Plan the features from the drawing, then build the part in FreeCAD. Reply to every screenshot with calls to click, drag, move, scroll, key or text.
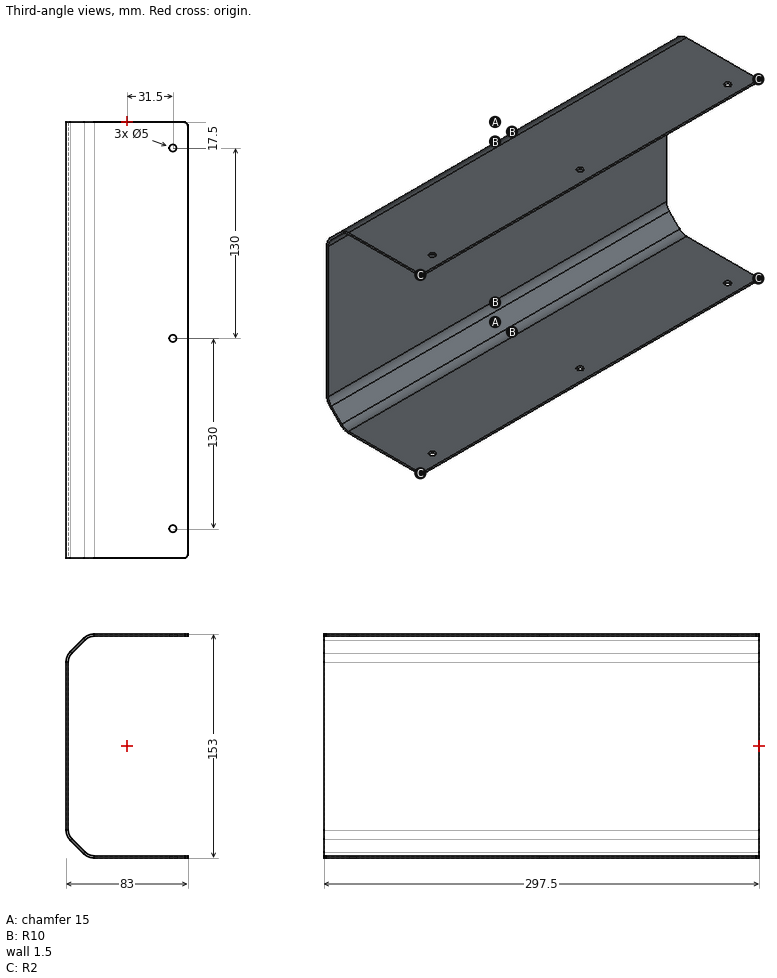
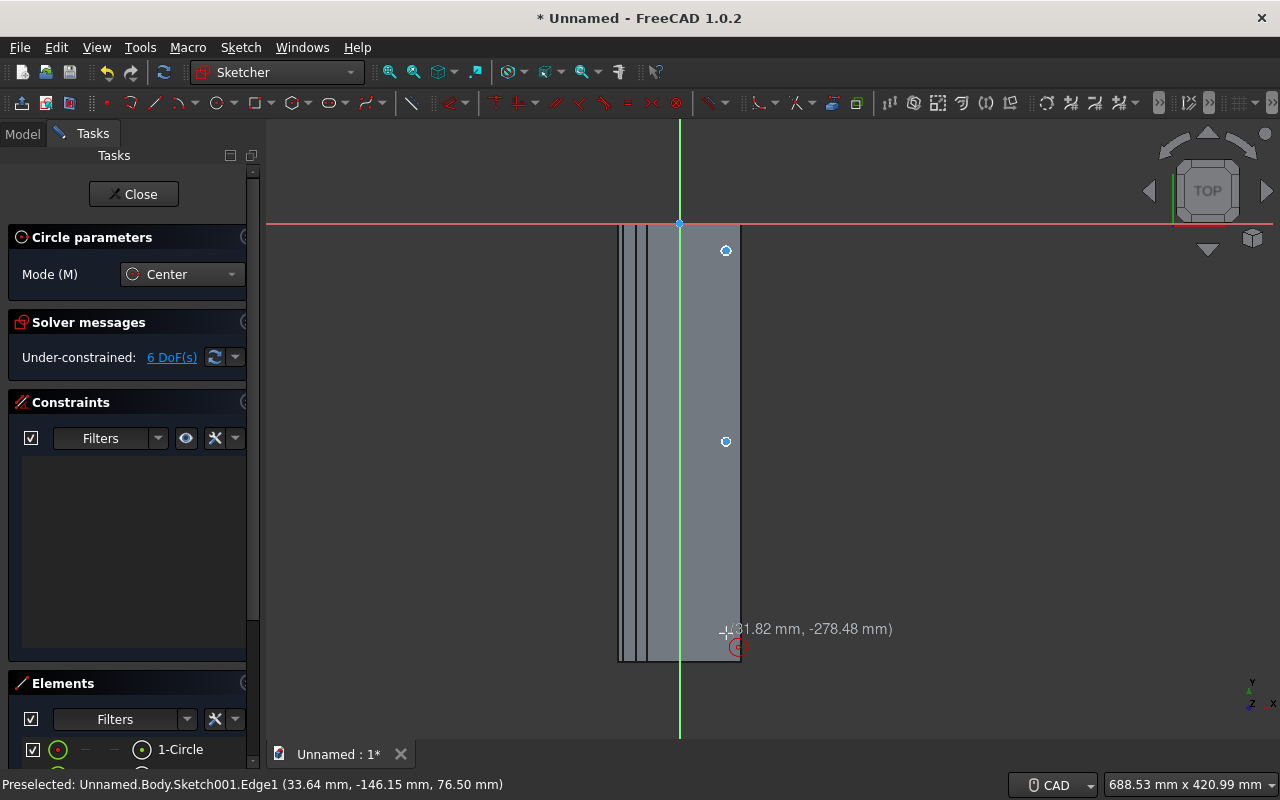
click(726, 632)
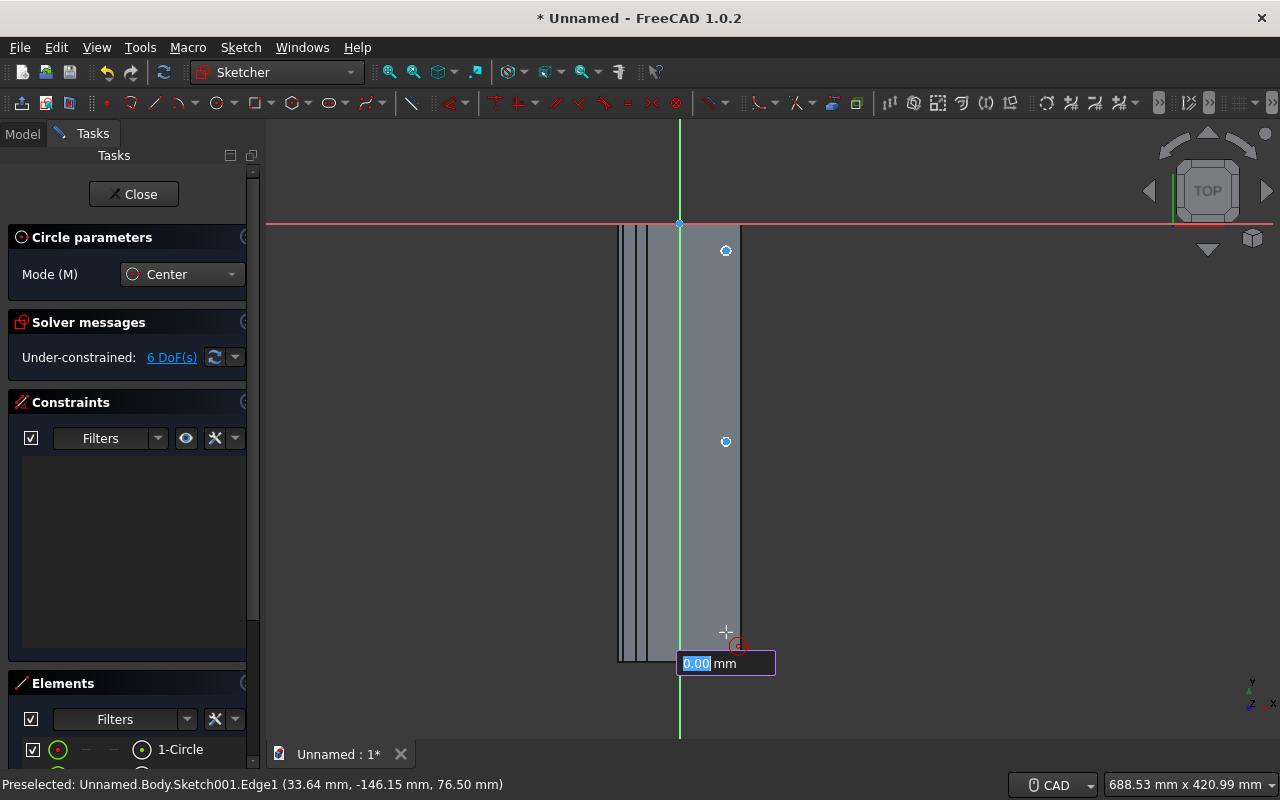
scroll(729, 630, up, 8)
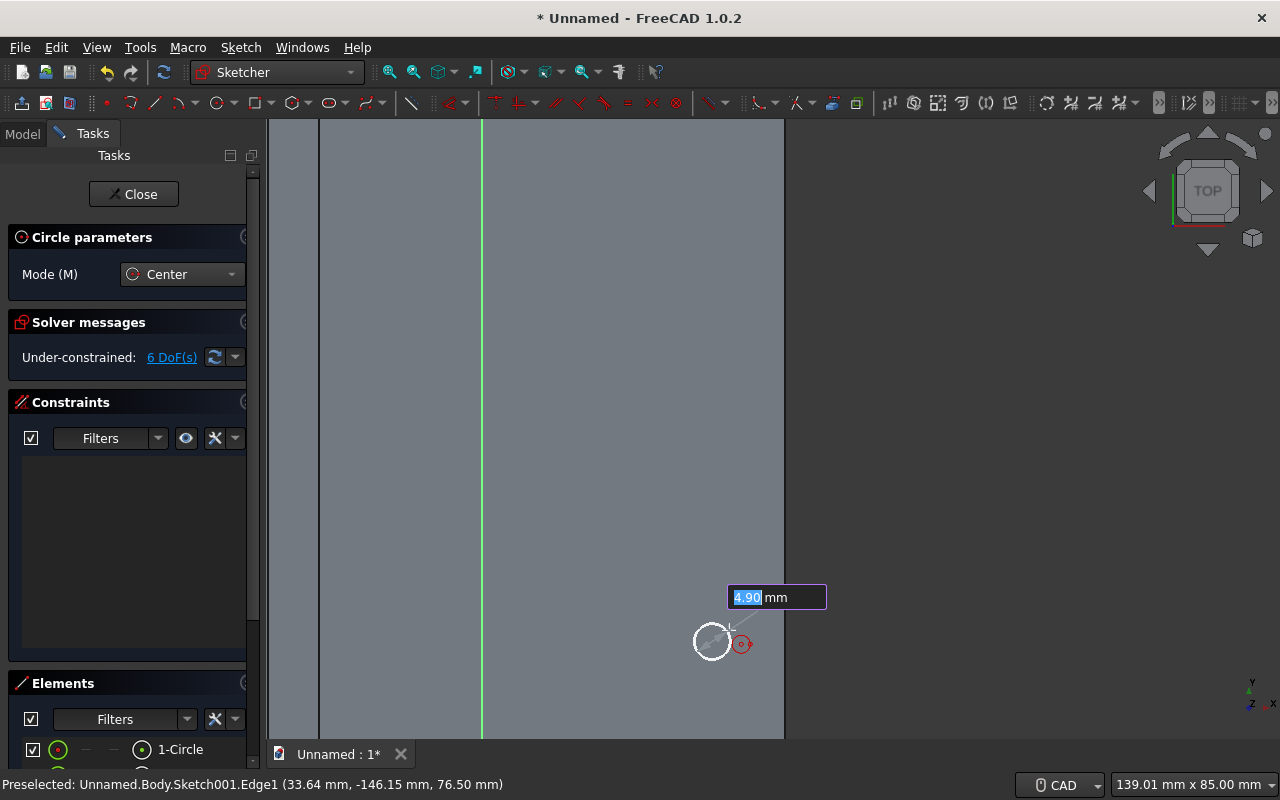
click(725, 626)
key(Escape)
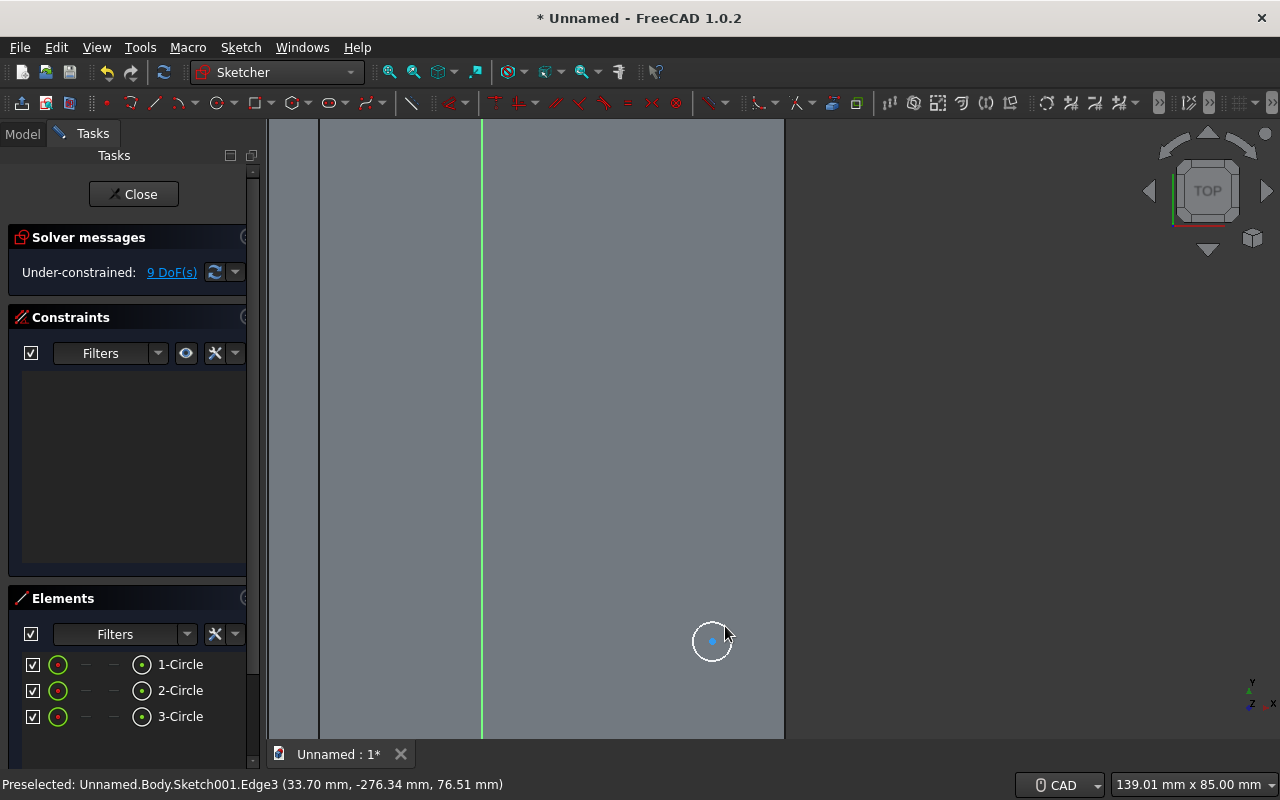
scroll(729, 630, down, 8)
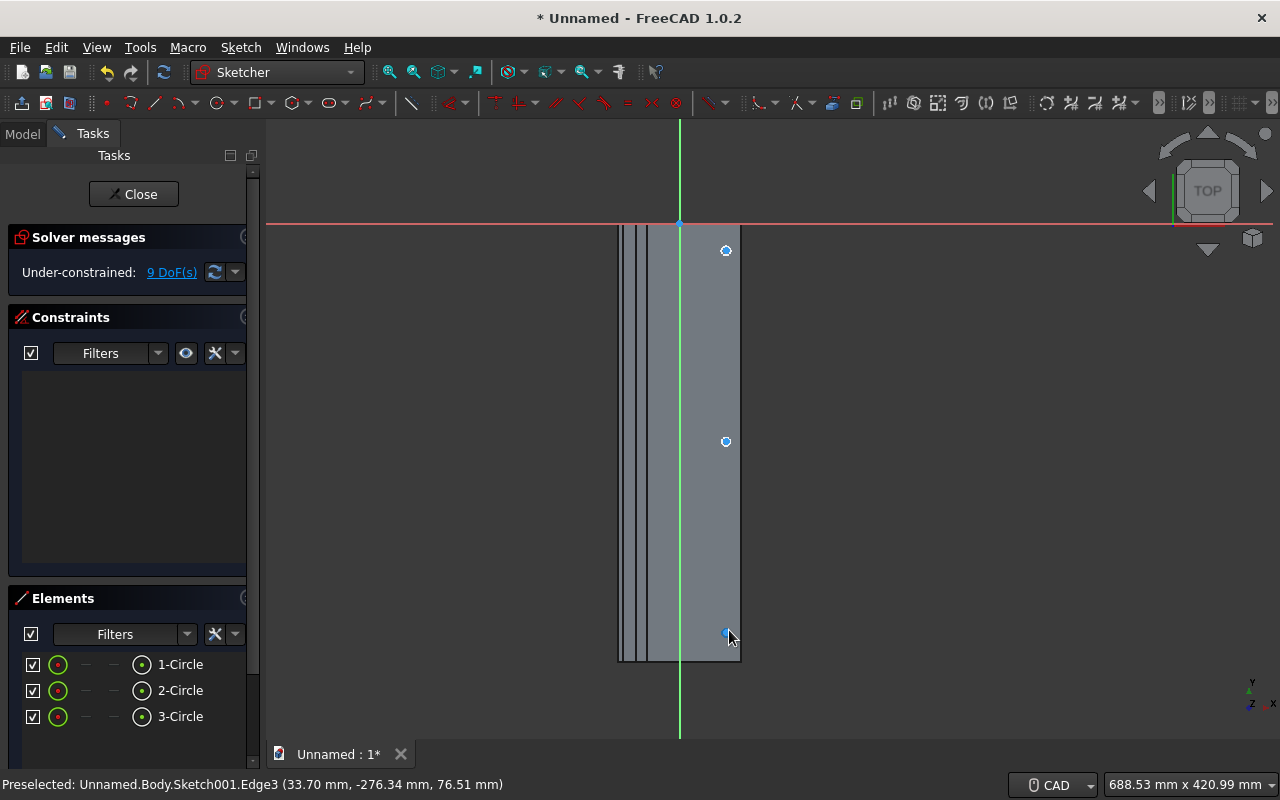
scroll(729, 248, up, 6)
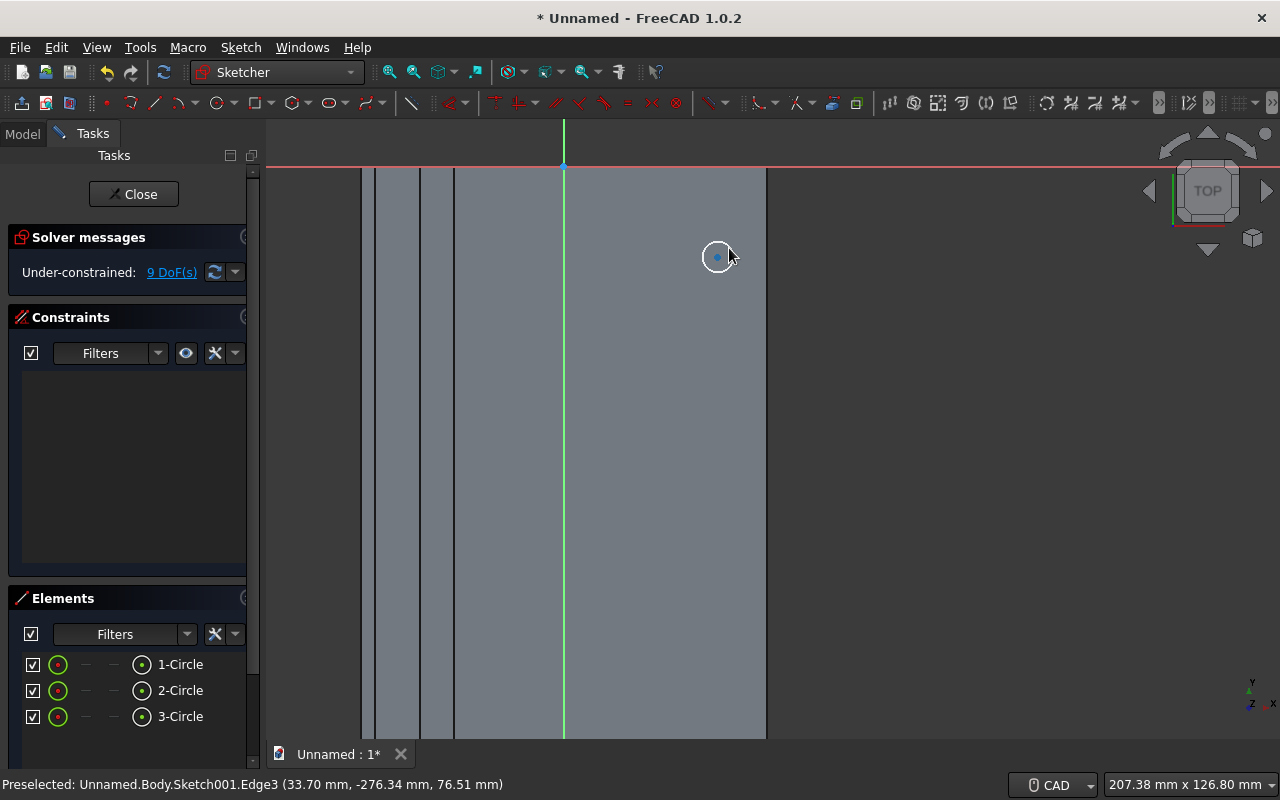
click(729, 246)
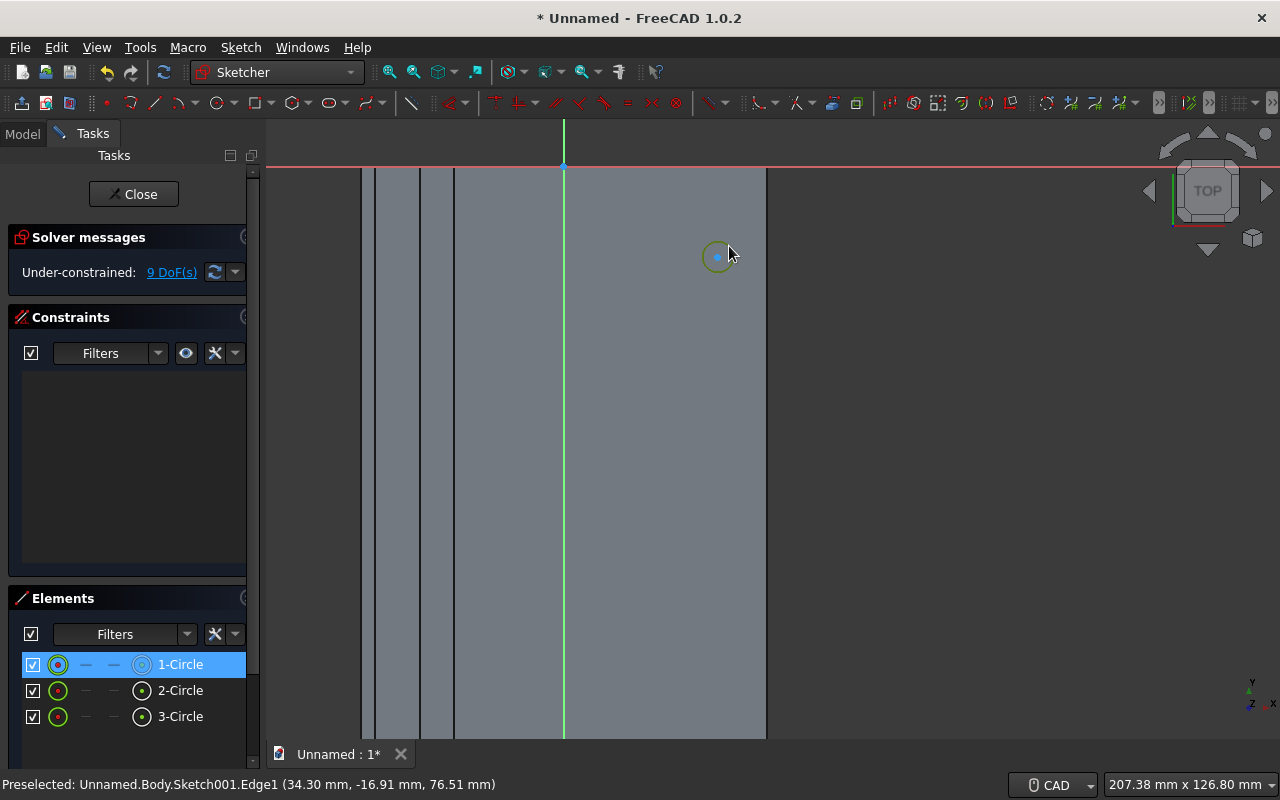
scroll(729, 247, down, 6)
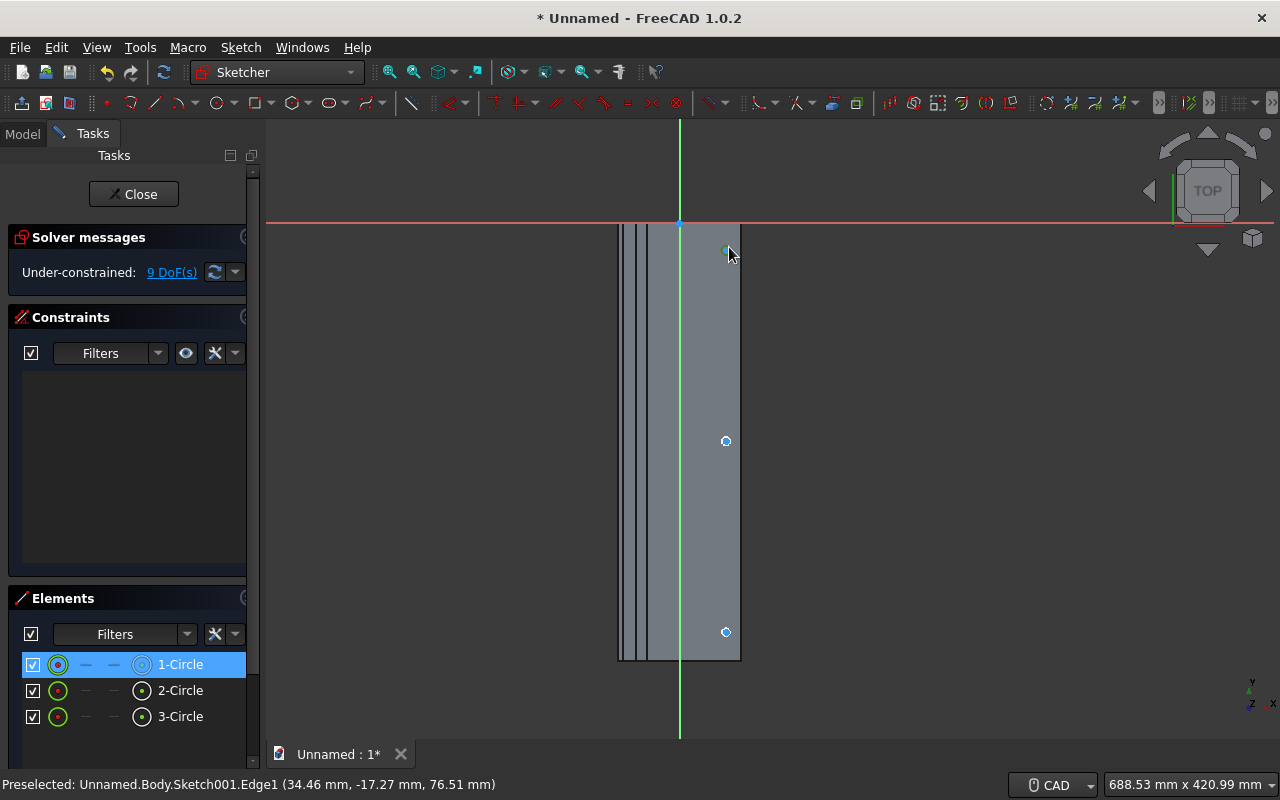
scroll(729, 438, up, 6)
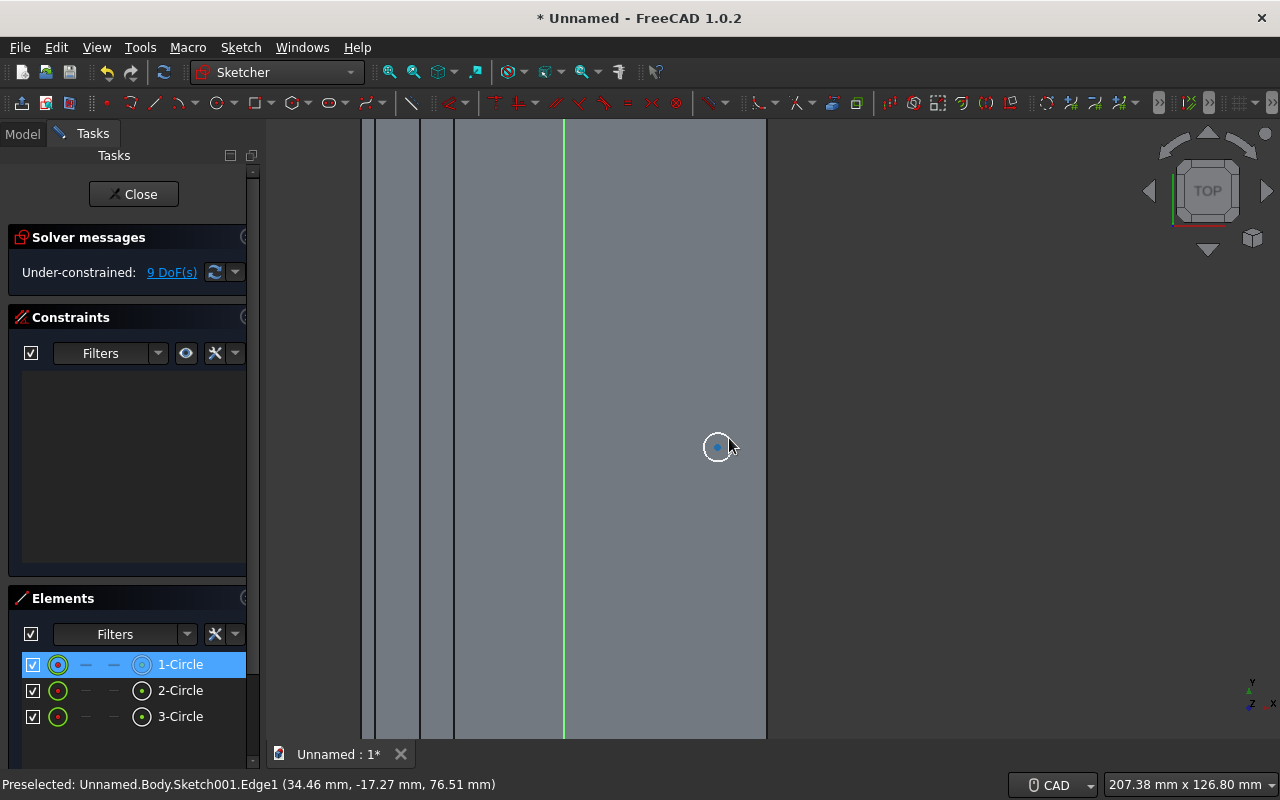
click(728, 437)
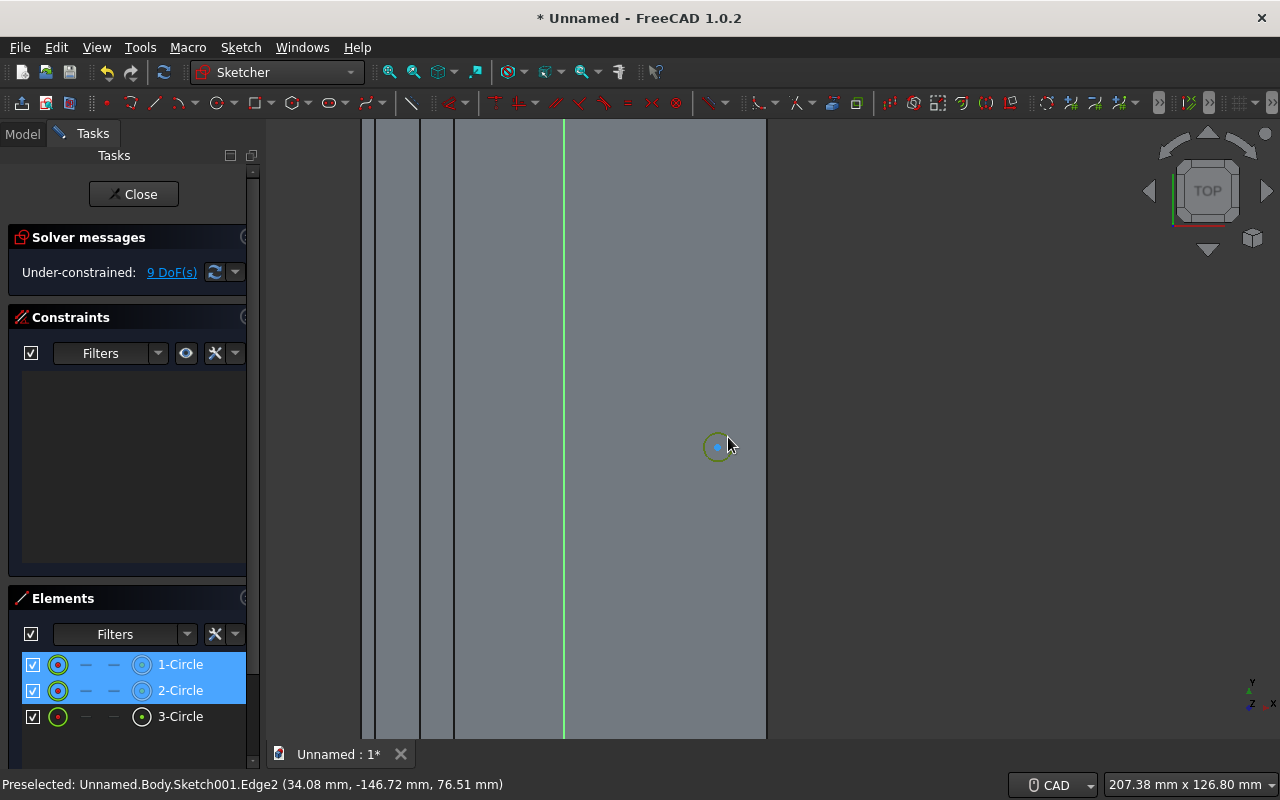
scroll(729, 438, down, 6)